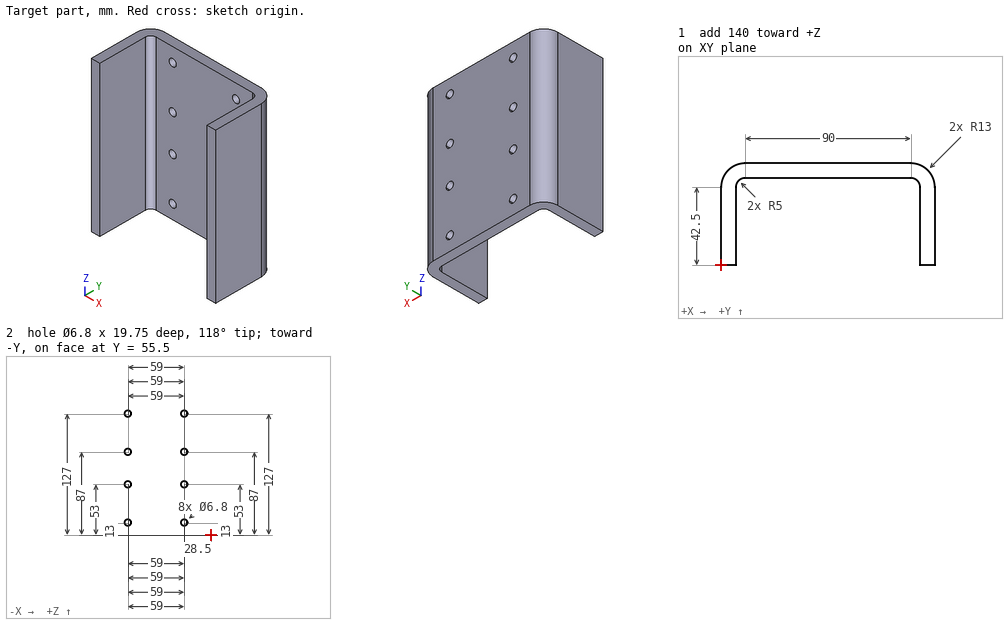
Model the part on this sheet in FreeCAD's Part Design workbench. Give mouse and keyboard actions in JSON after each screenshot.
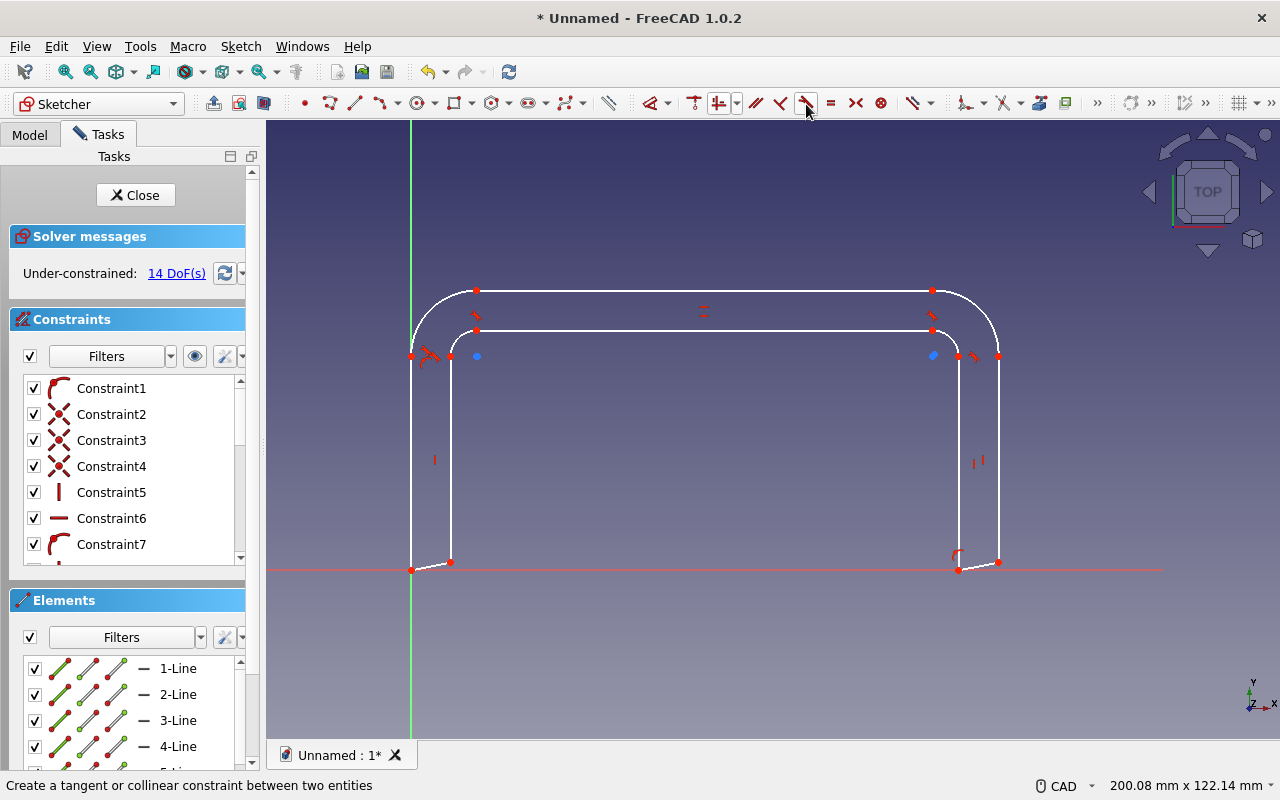
{"action": "left_click", "coordinate": [999, 501]}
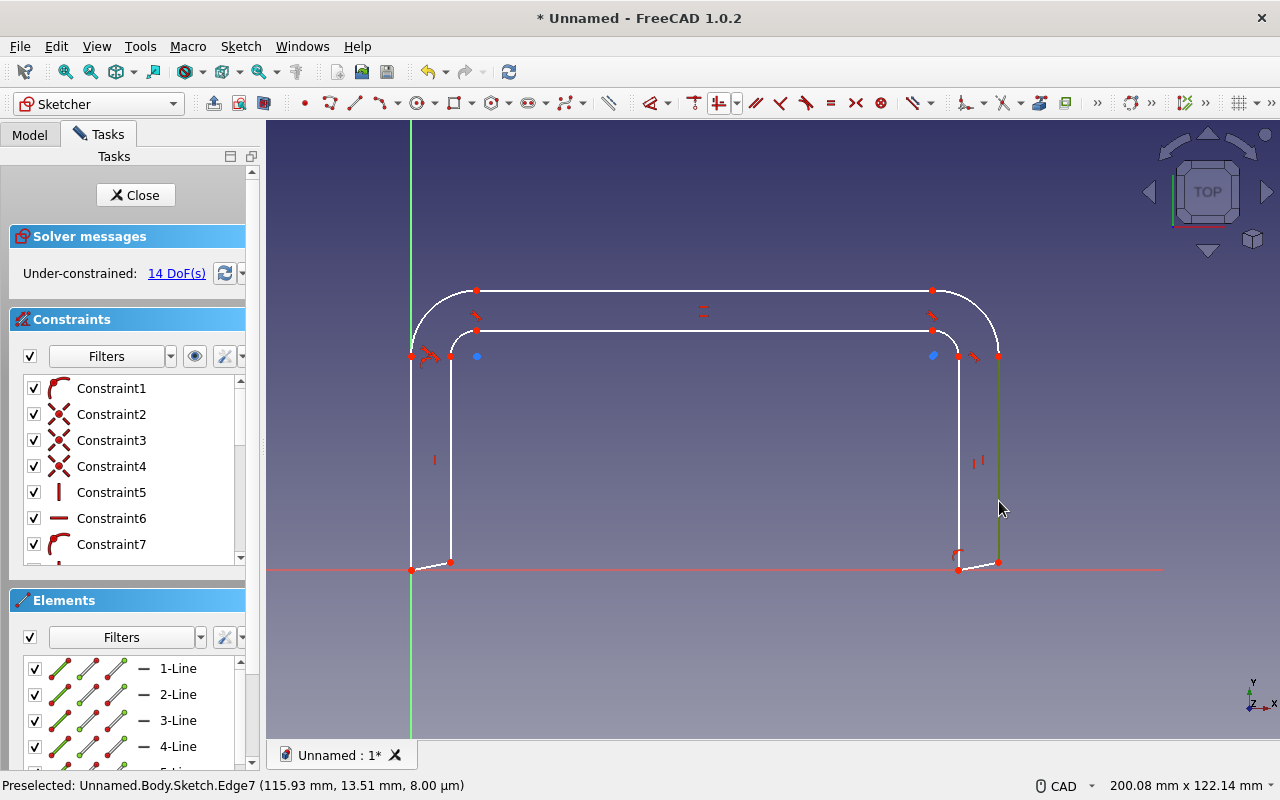
{"action": "left_click", "coordinate": [992, 326]}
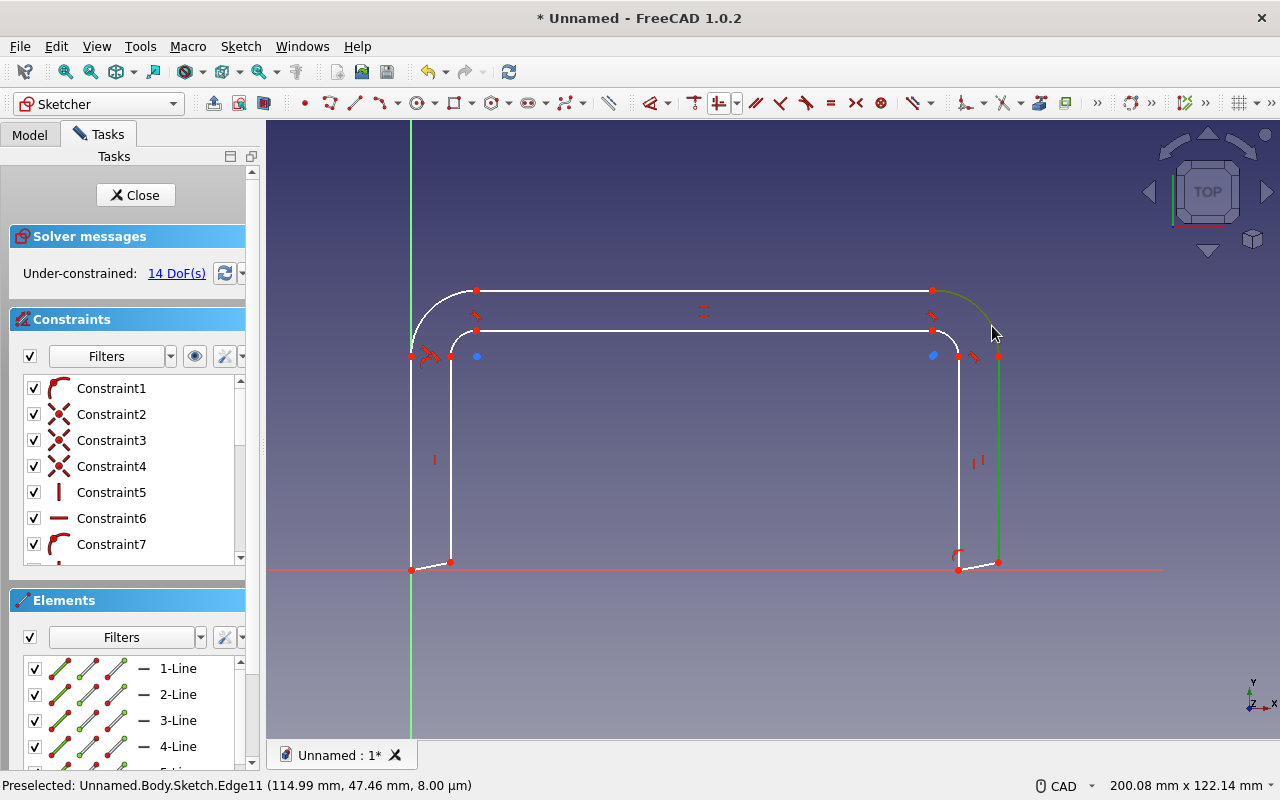
{"action": "key", "text": "t"}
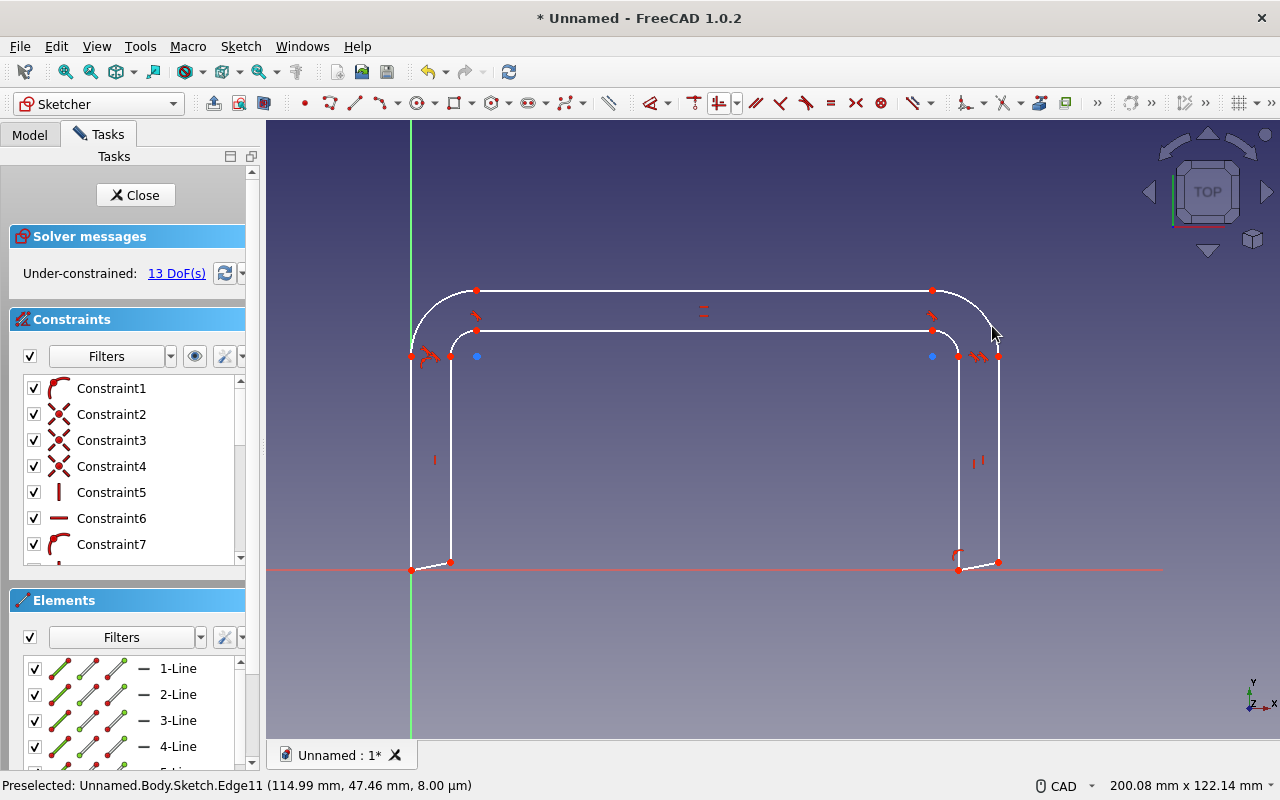
{"action": "left_click", "coordinate": [796, 291]}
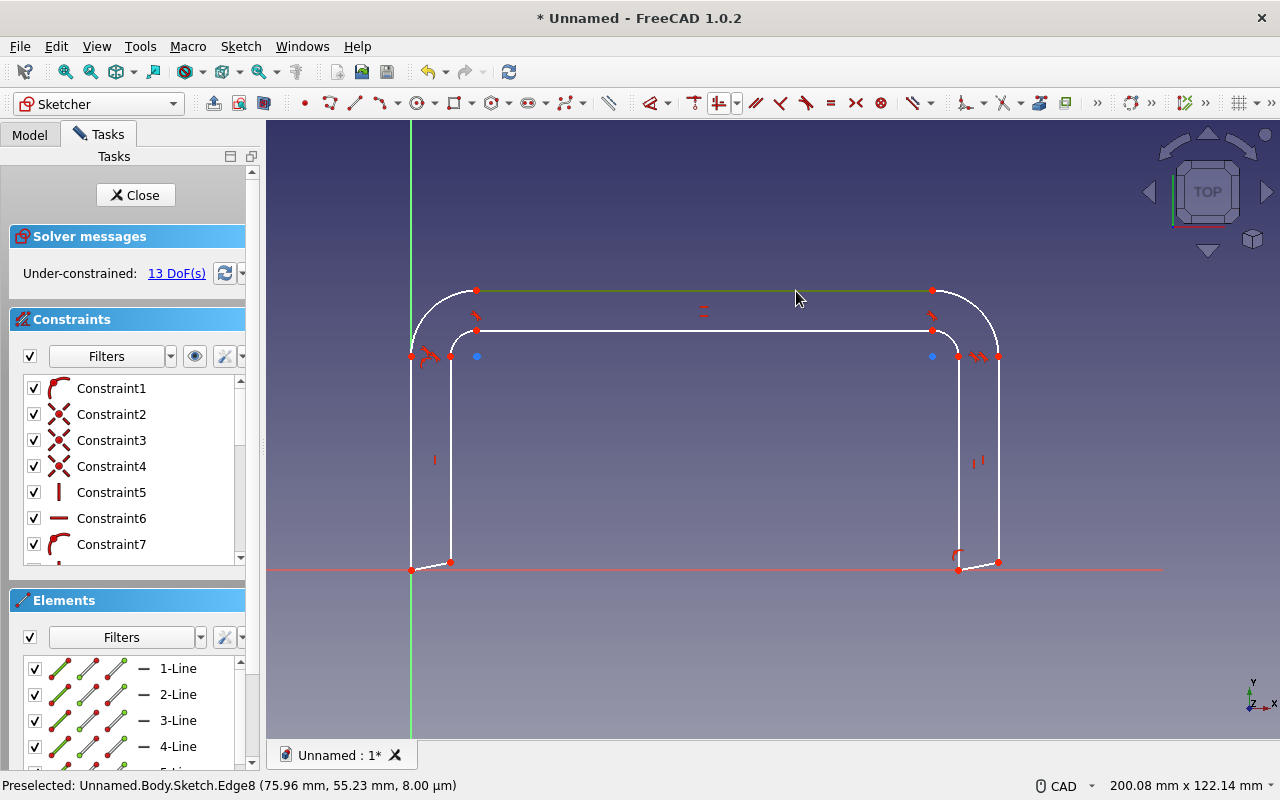
{"action": "left_click", "coordinate": [991, 327]}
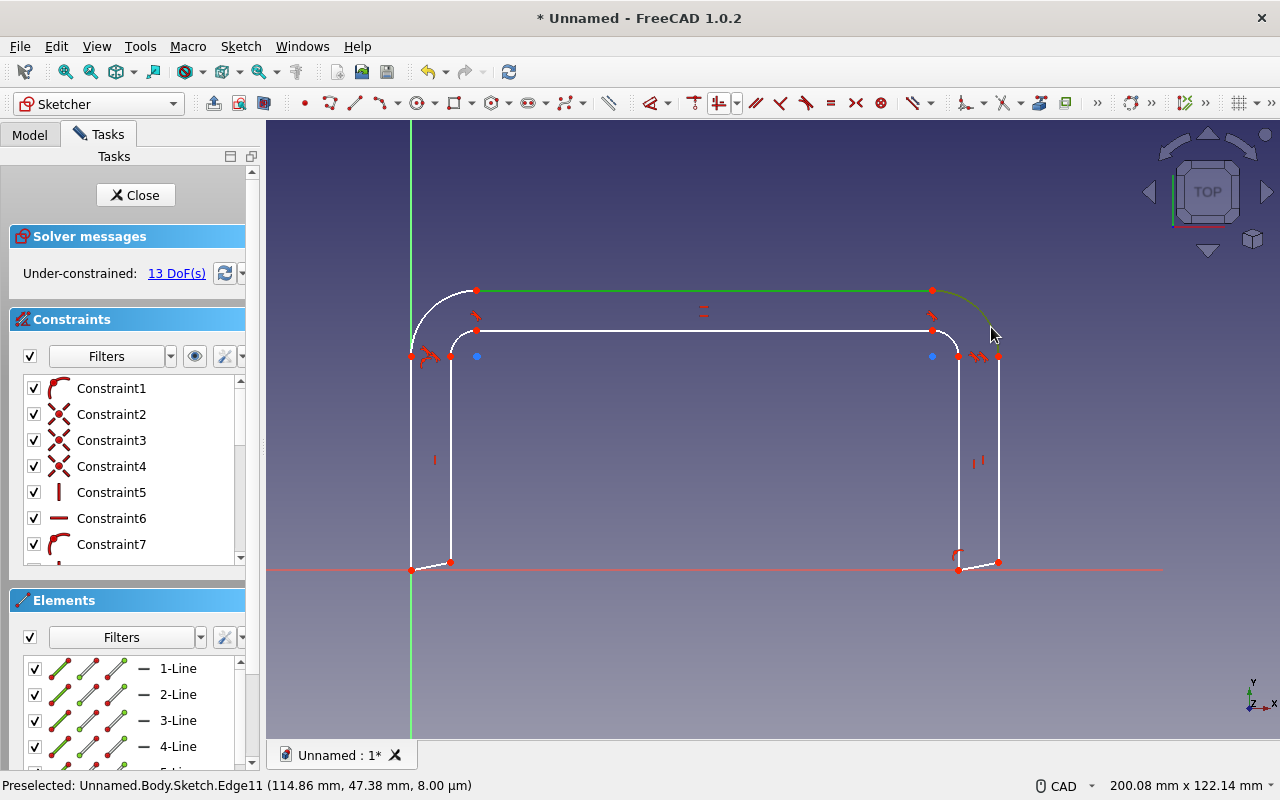
{"action": "key", "text": "t"}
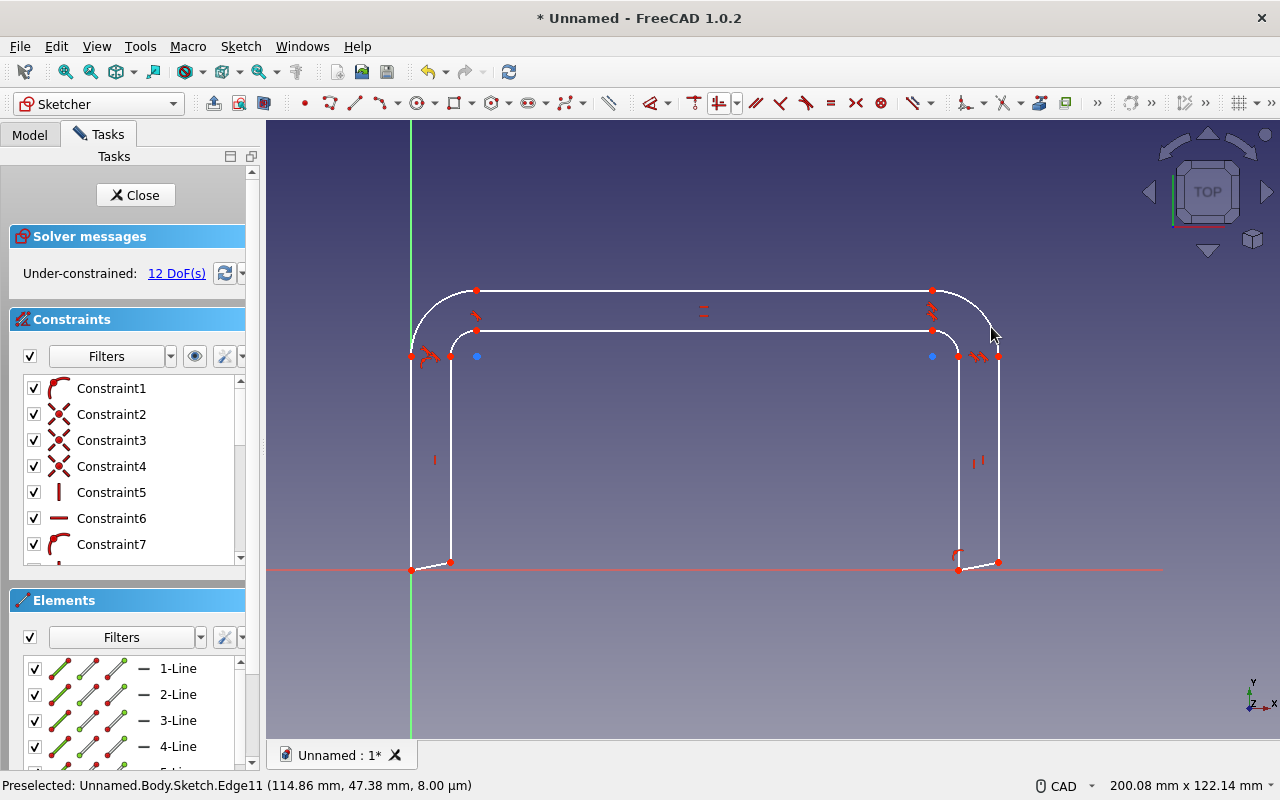
{"action": "left_click", "coordinate": [796, 291]}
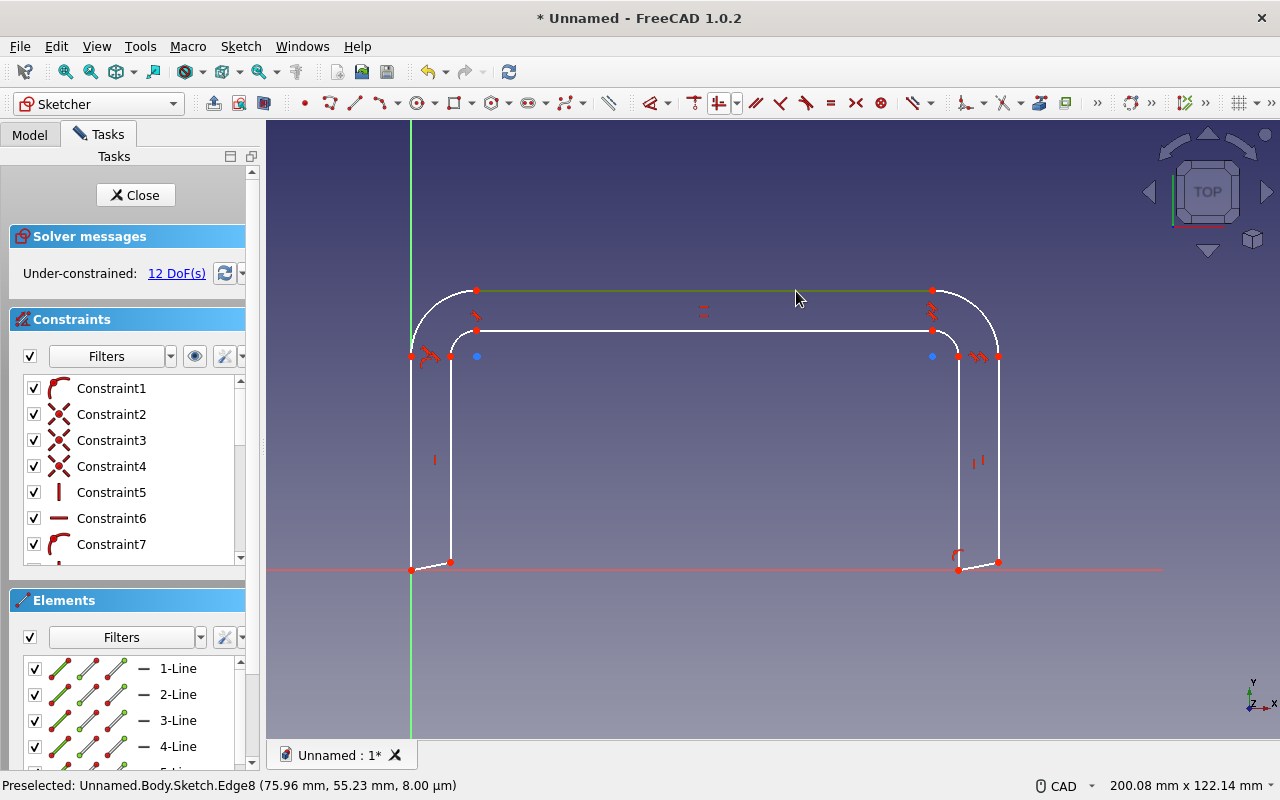
{"action": "left_click", "coordinate": [447, 298]}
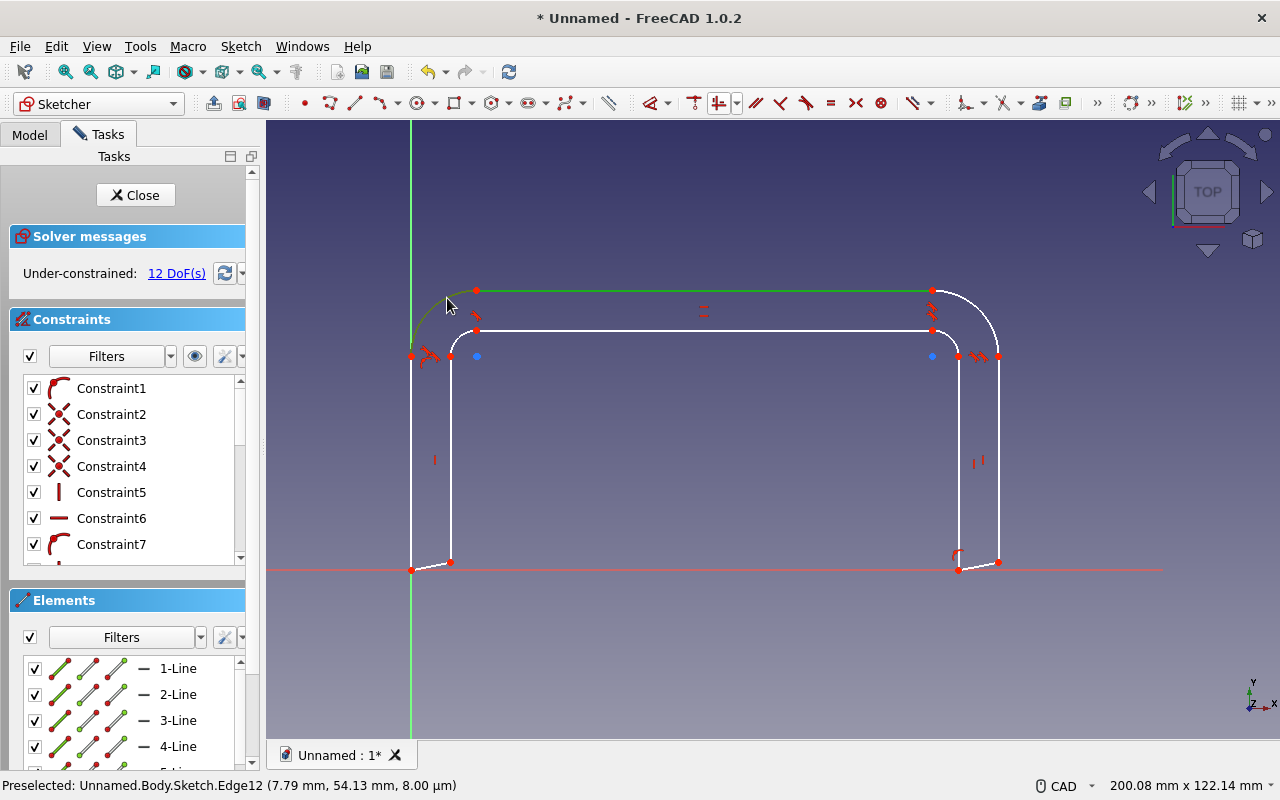
{"action": "key", "text": "t"}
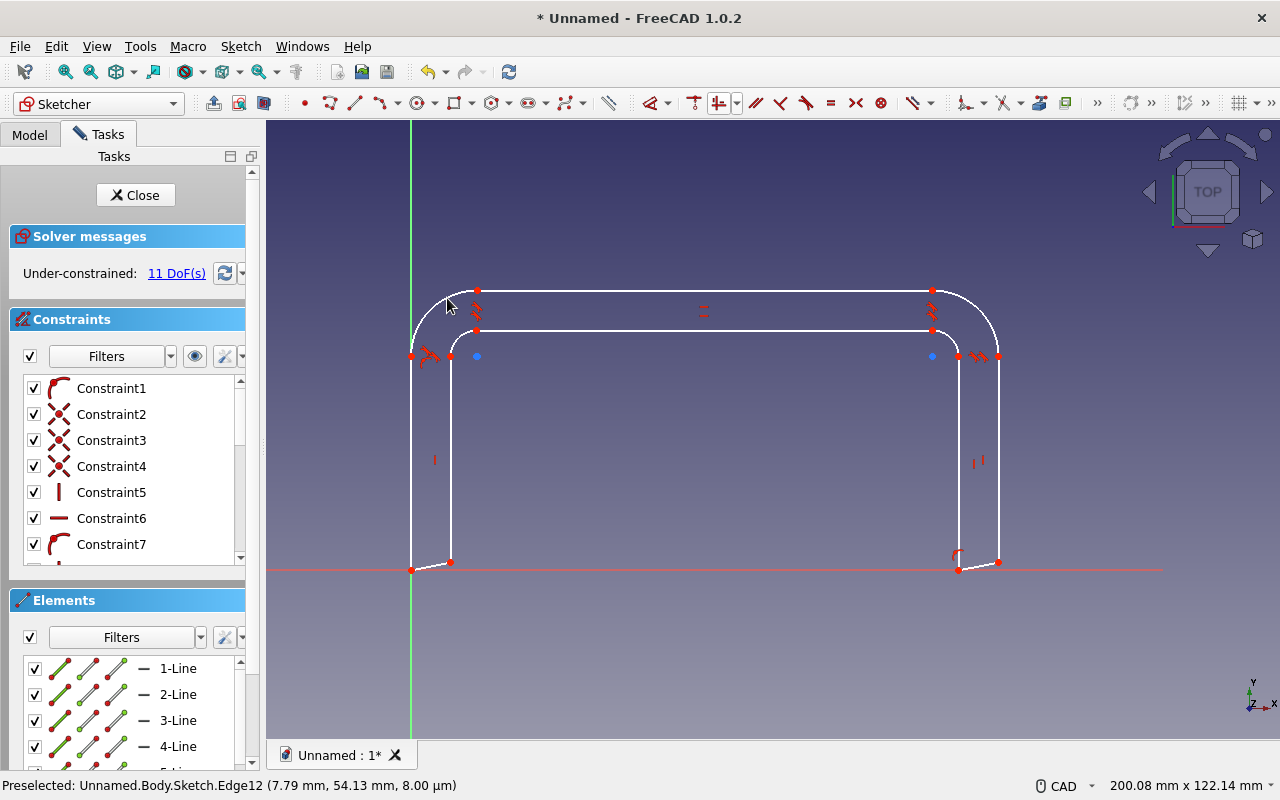
{"action": "left_click", "coordinate": [423, 568]}